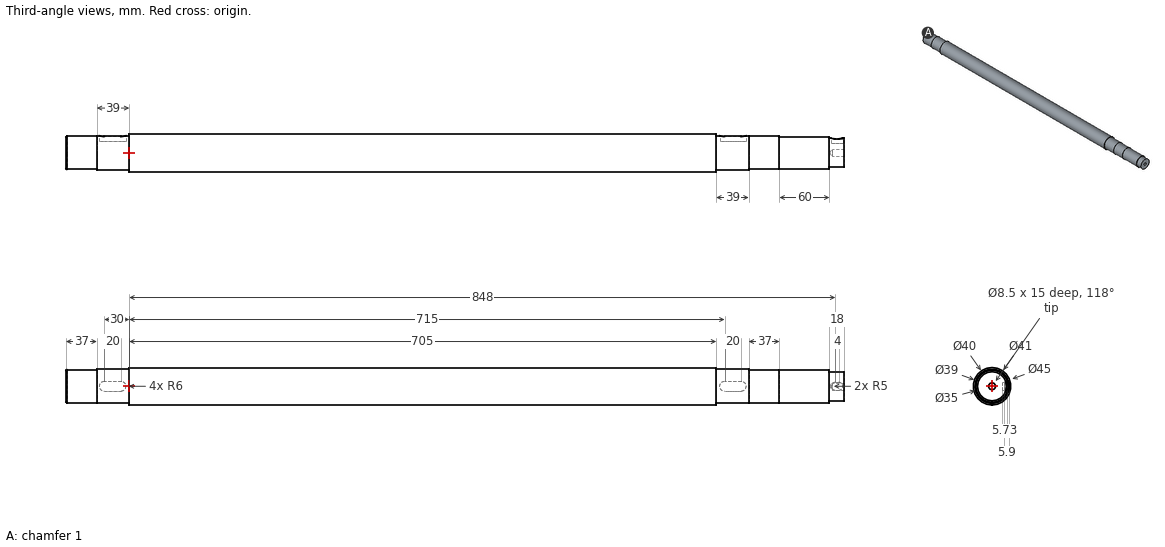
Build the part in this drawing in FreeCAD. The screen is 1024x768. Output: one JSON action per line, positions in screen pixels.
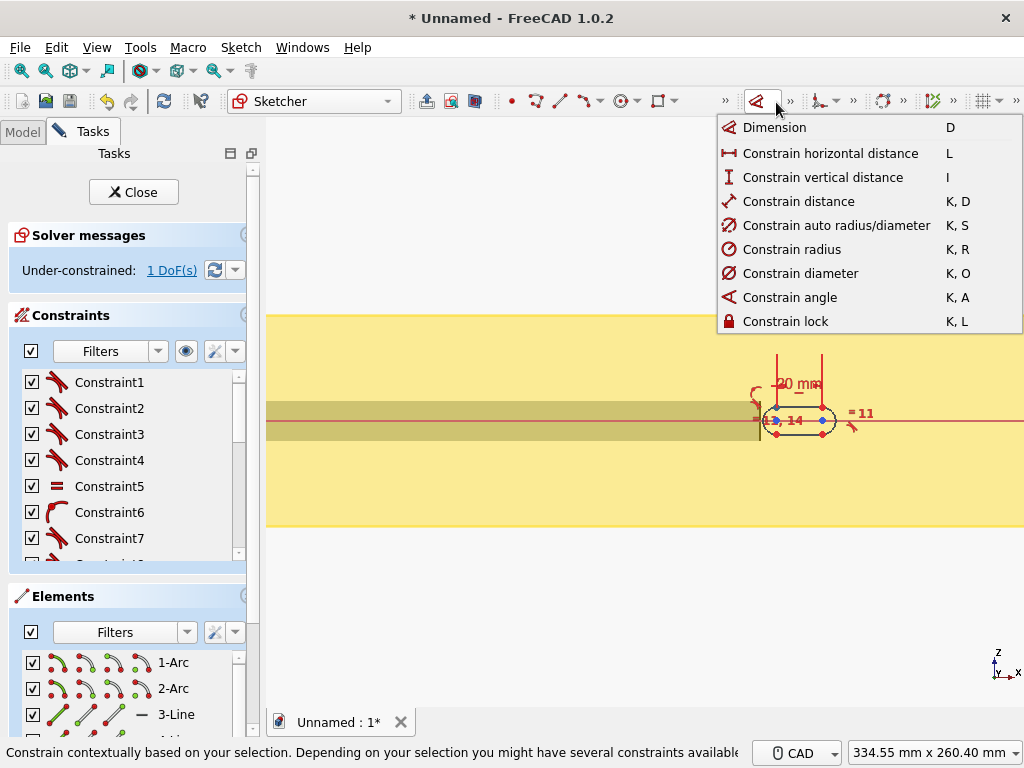
{"action": "left_click", "coordinate": [870, 153]}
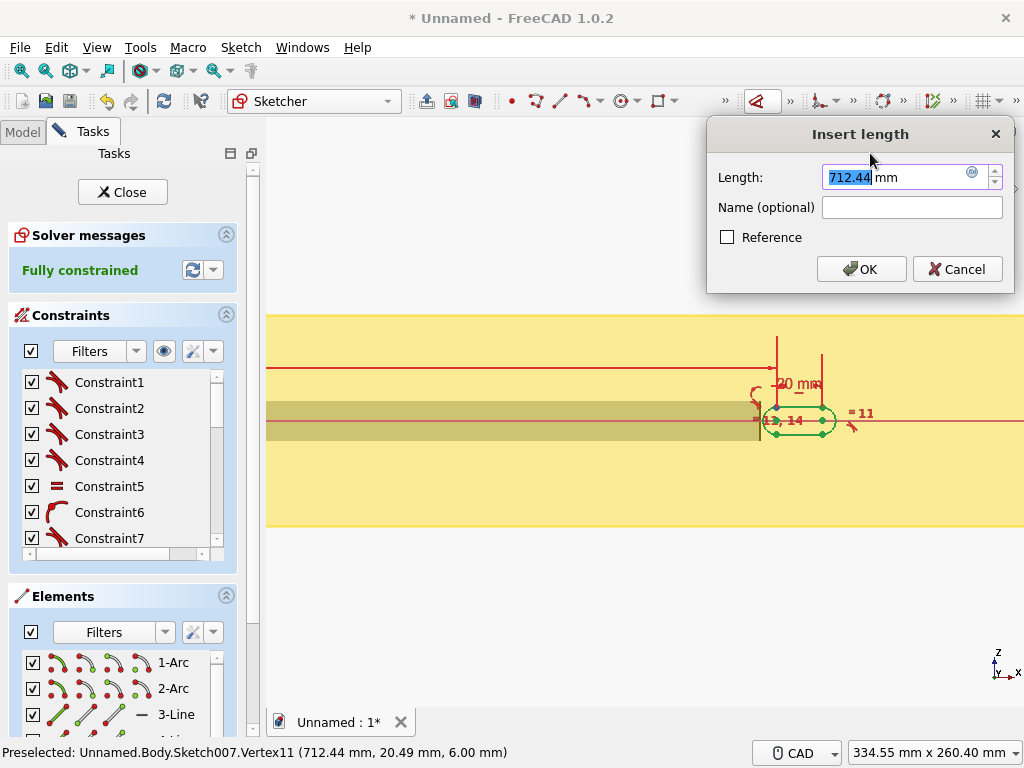
{"action": "type", "text": "715"}
{"action": "key", "text": "Return"}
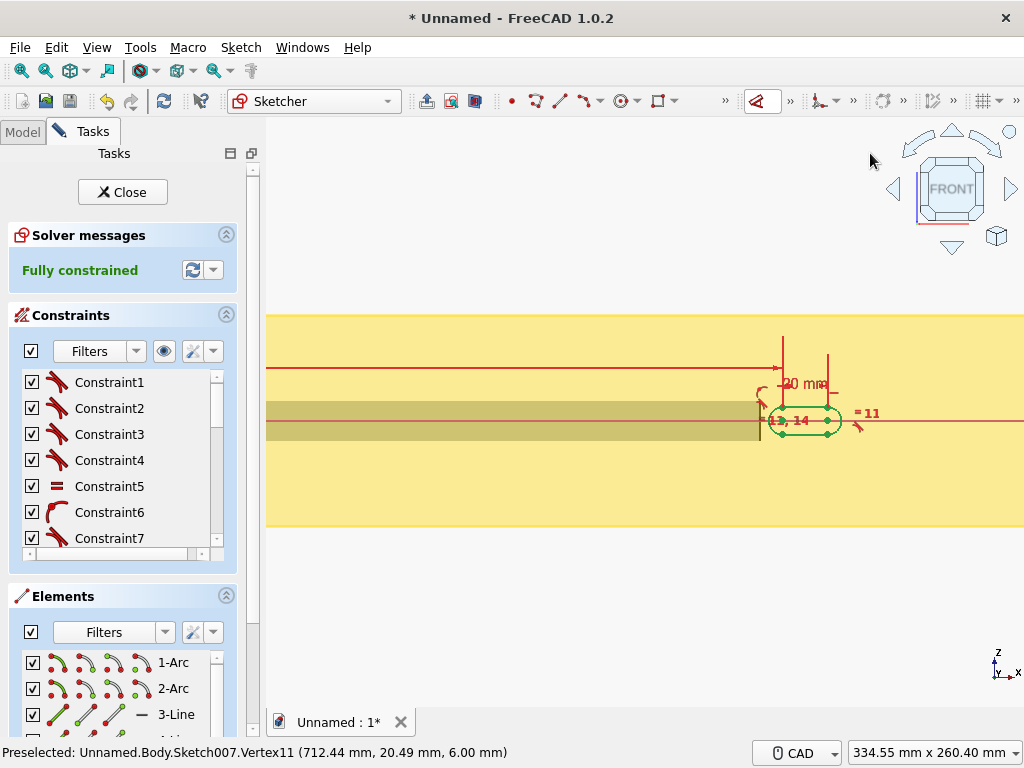
{"action": "left_click", "coordinate": [123, 192]}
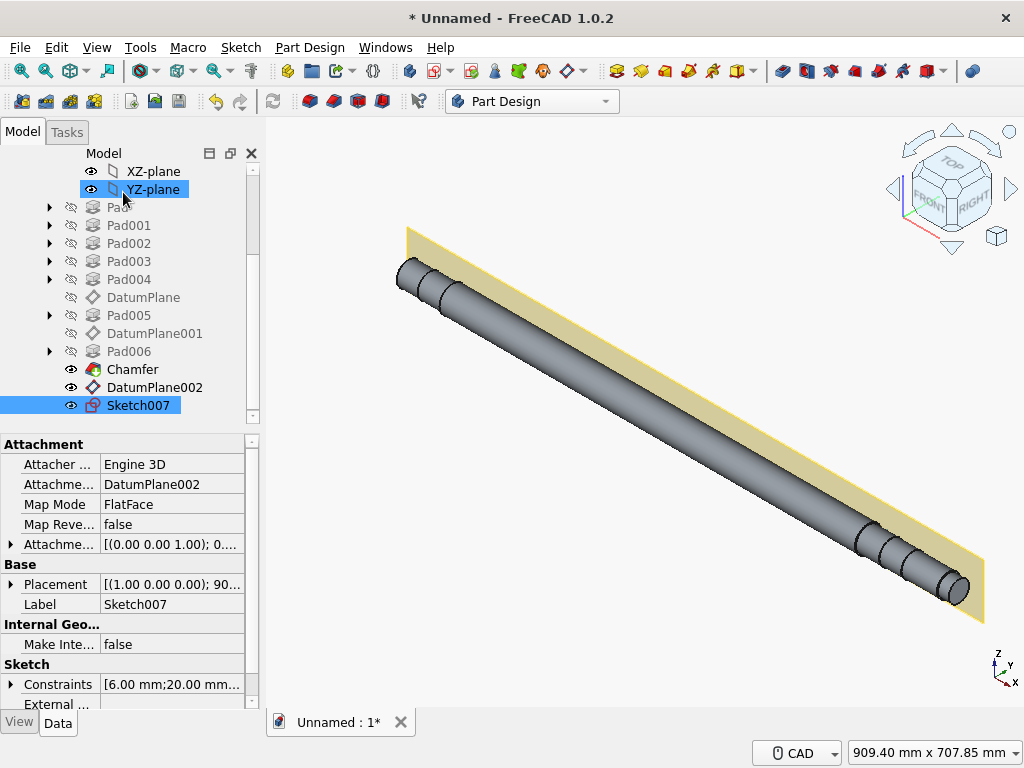
{"action": "left_click", "coordinate": [784, 72]}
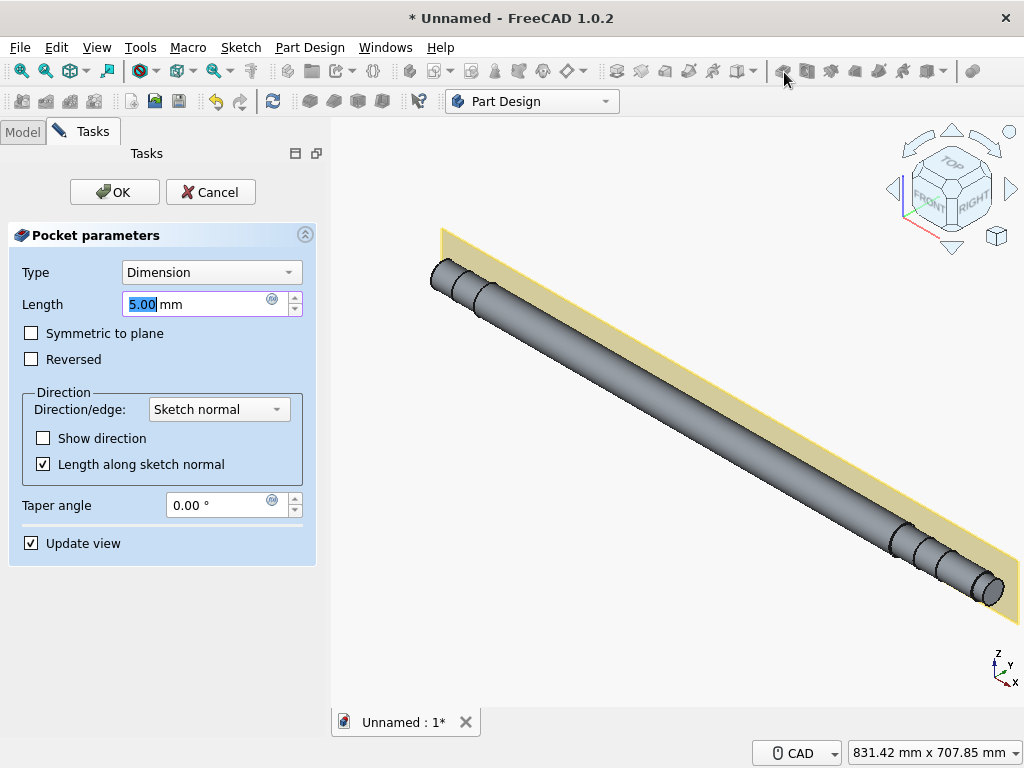
{"action": "type", "text": "5.9"}
{"action": "key", "text": "Tab"}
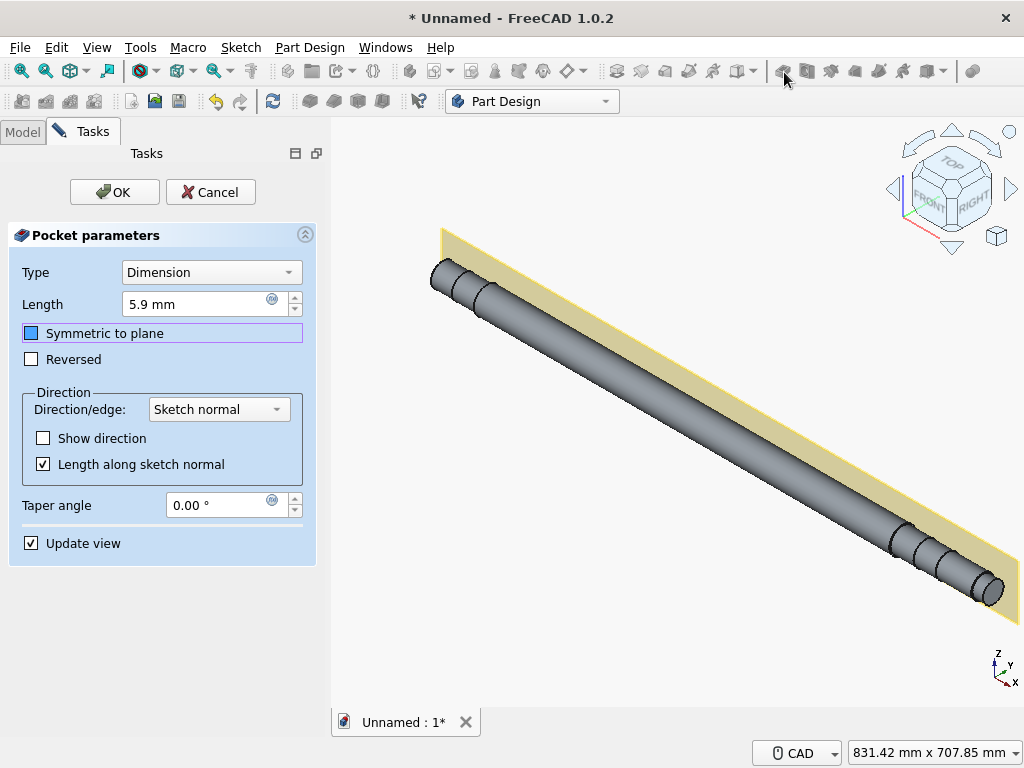
{"action": "left_click", "coordinate": [30, 359]}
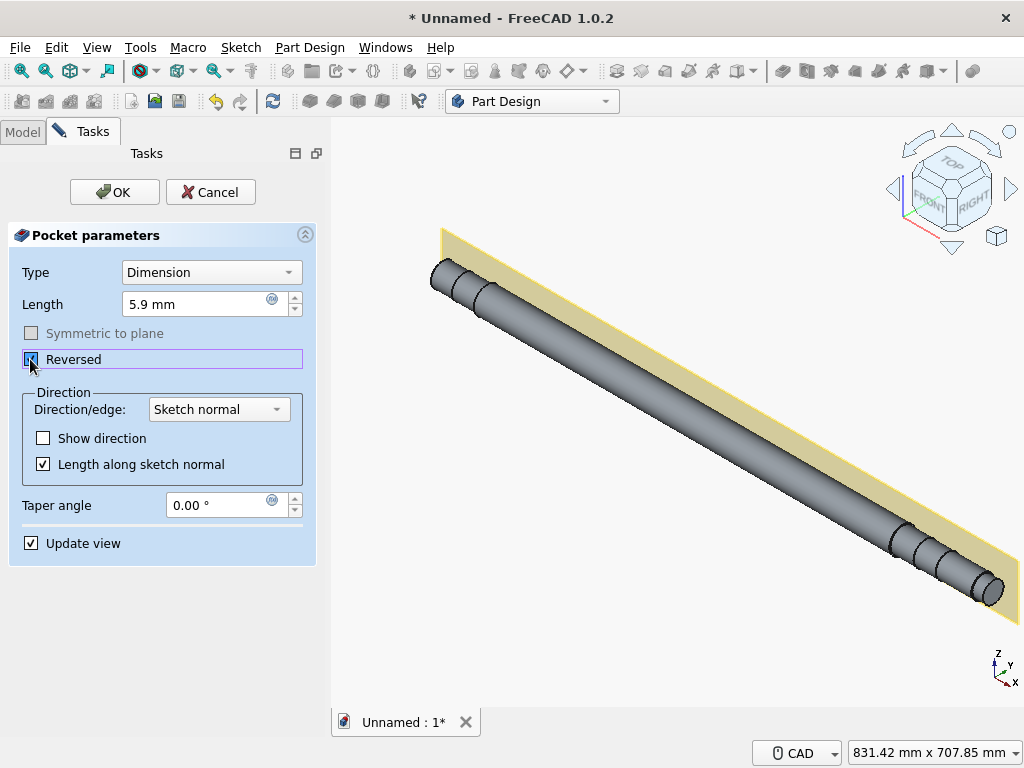
{"action": "left_click", "coordinate": [115, 192]}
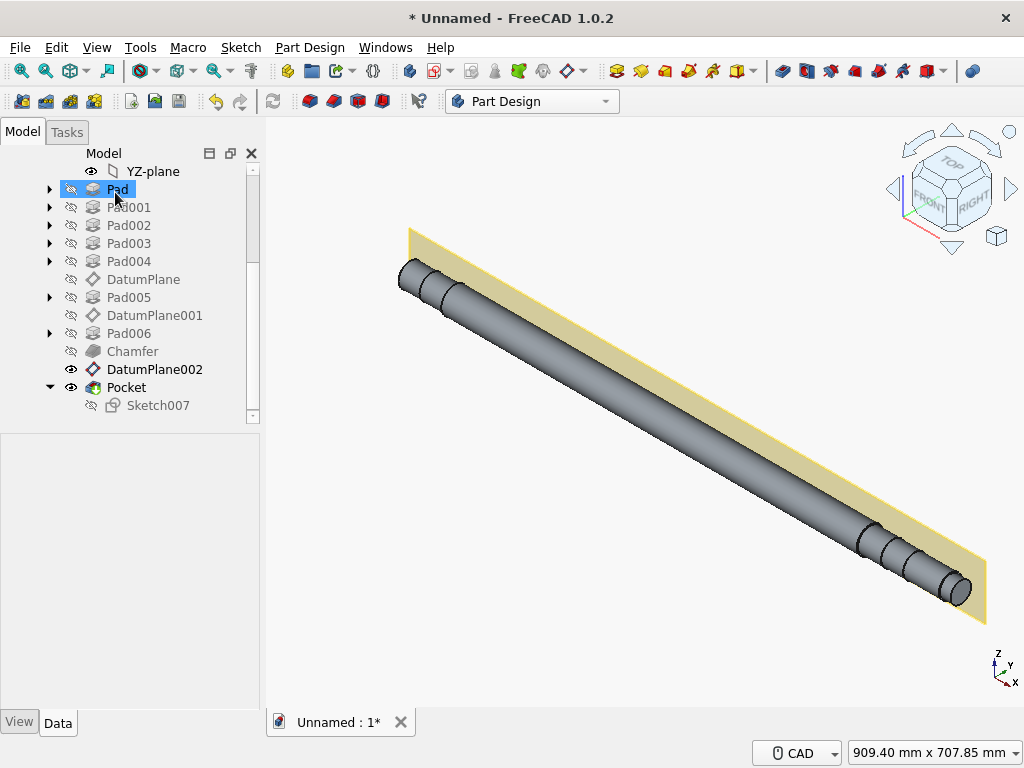
{"action": "left_click", "coordinate": [116, 369]}
{"action": "key", "text": "space"}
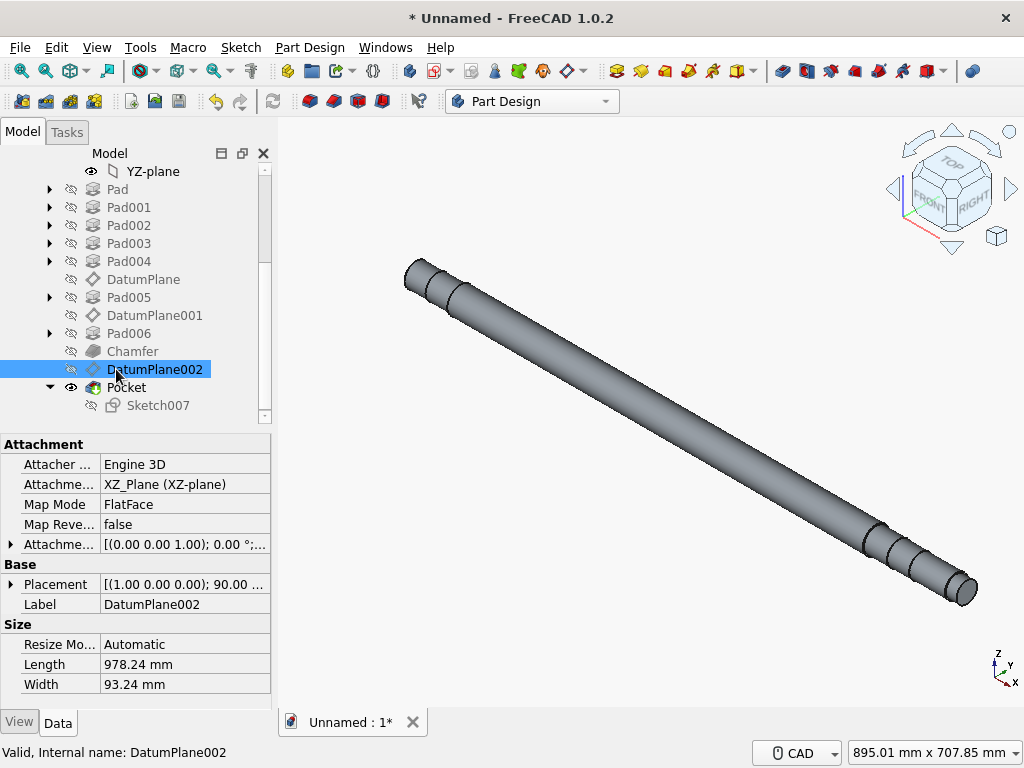
{"action": "scroll", "coordinate": [160, 293], "scroll_direction": "down", "scroll_amount": 3}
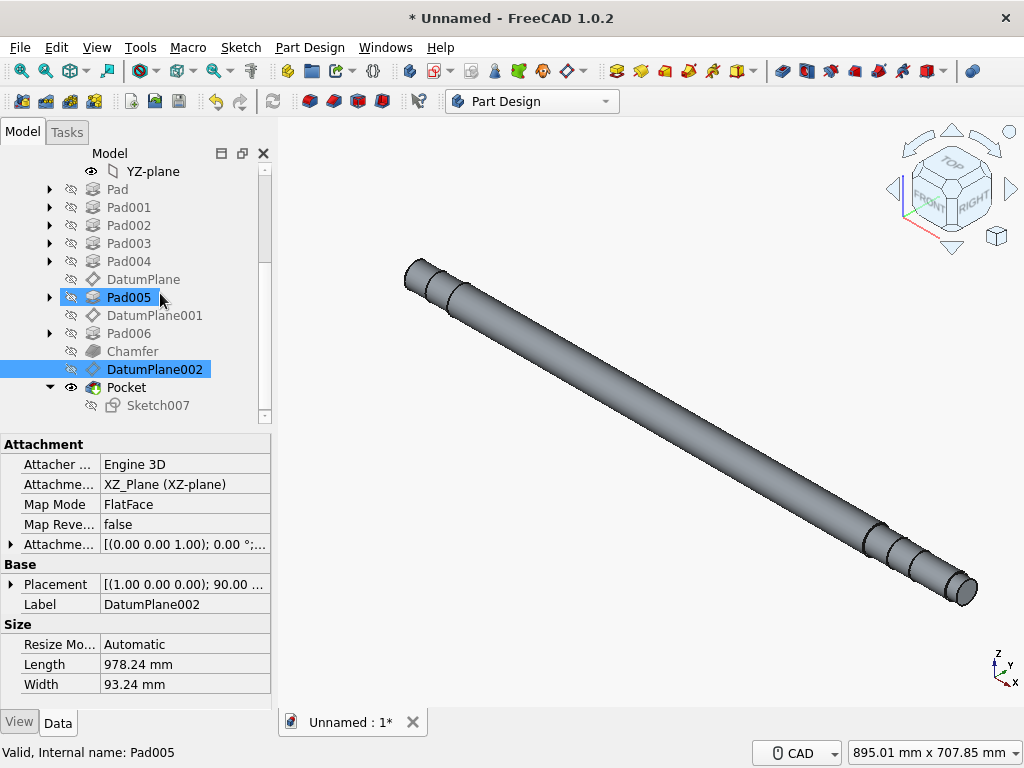
{"action": "scroll", "coordinate": [160, 293], "scroll_direction": "up", "scroll_amount": 15}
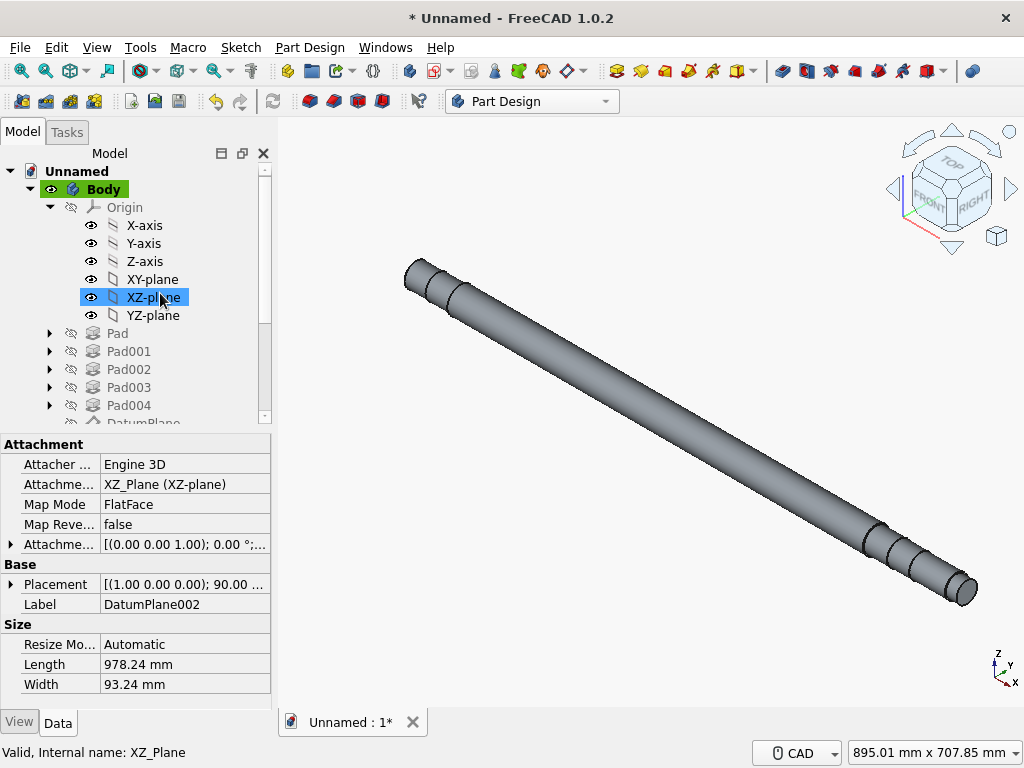
{"action": "left_click", "coordinate": [136, 297]}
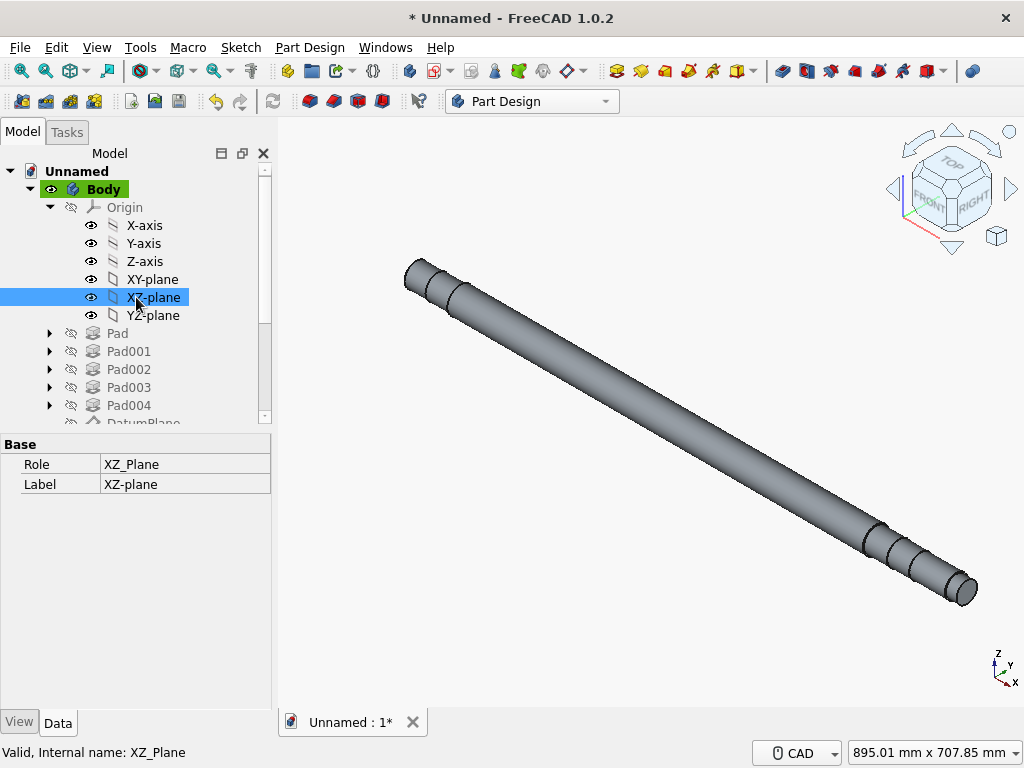
{"action": "left_click", "coordinate": [568, 72]}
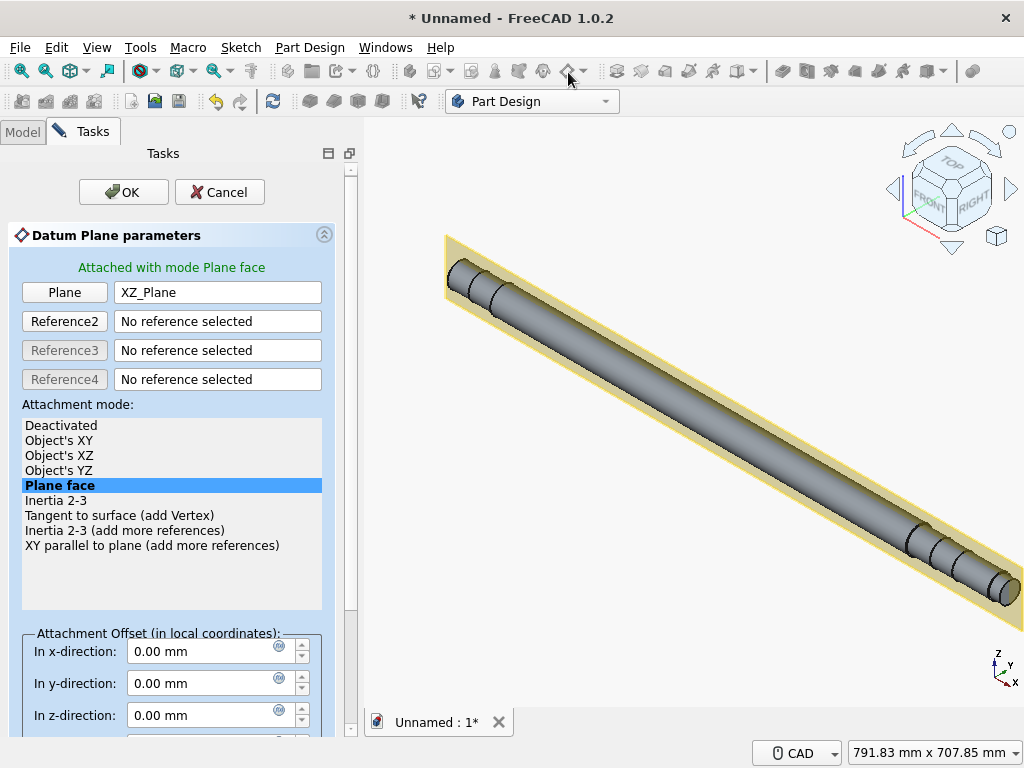
{"action": "triple_click", "coordinate": [210, 715]}